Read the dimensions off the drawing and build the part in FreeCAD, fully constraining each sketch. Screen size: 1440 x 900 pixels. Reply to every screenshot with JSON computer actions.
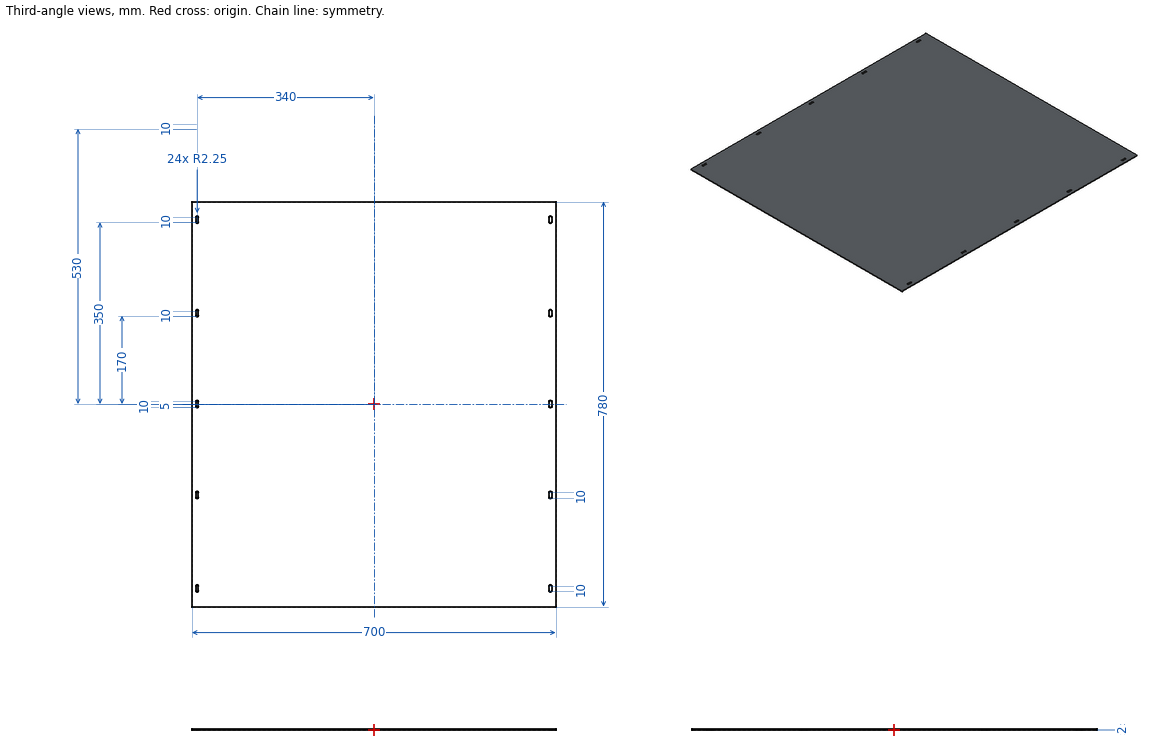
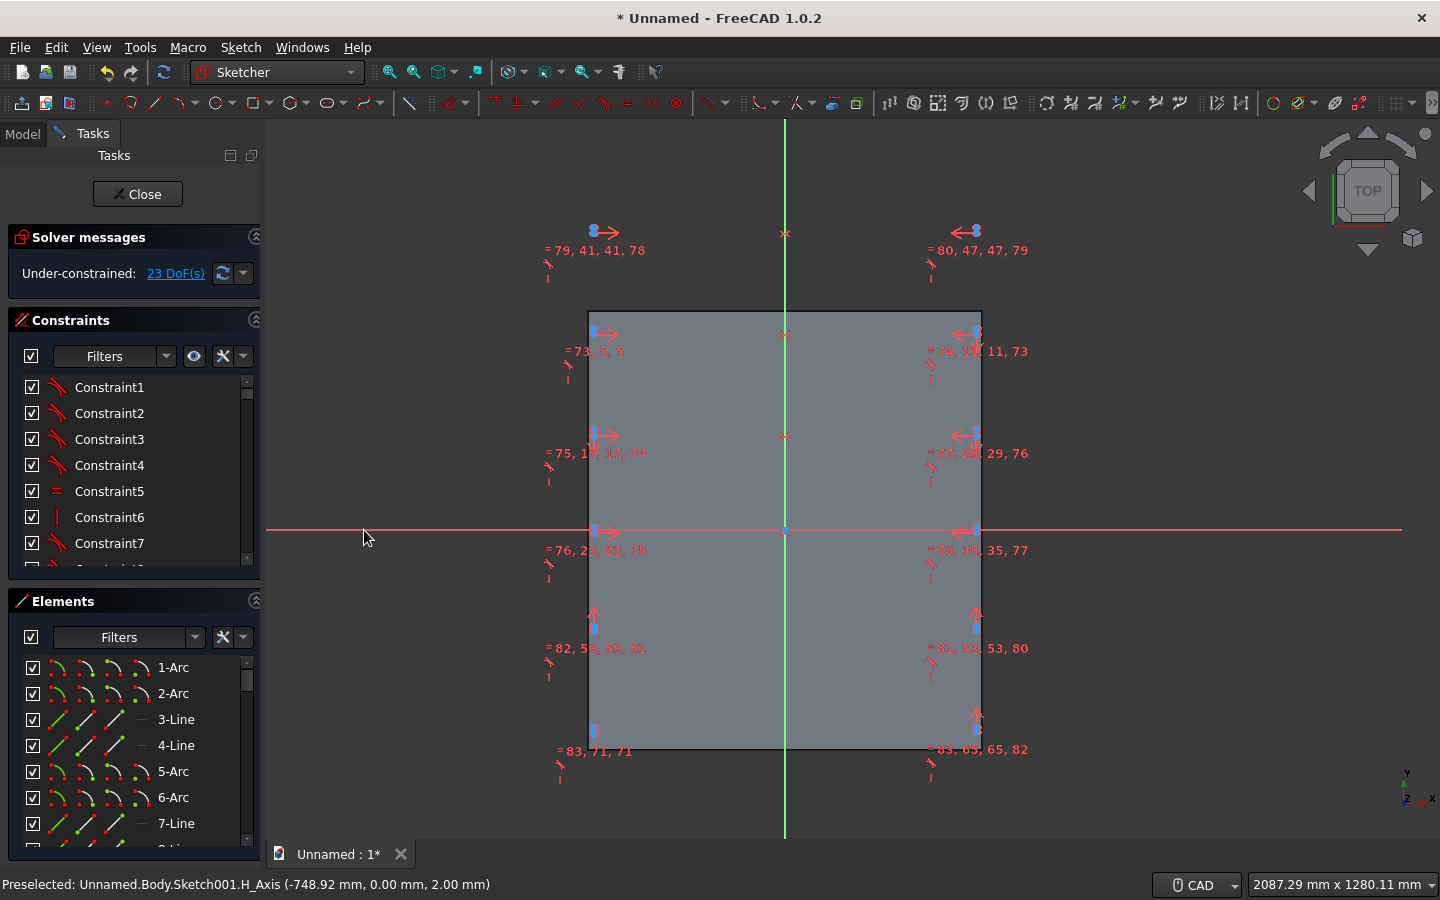
{"action": "scroll", "coordinate": [594, 328], "scroll_direction": "up", "scroll_amount": 12}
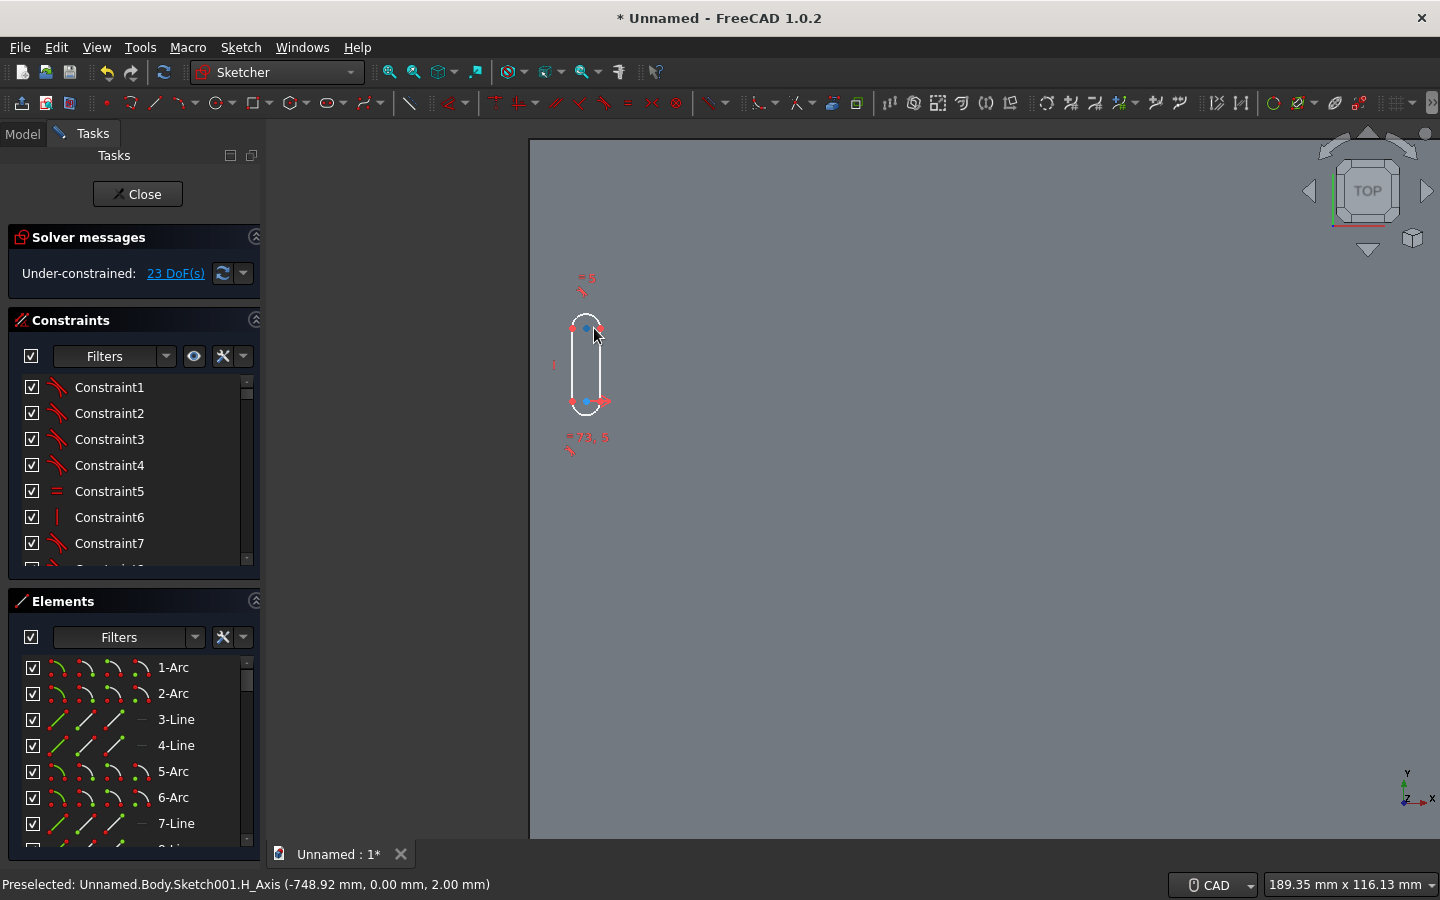
{"action": "left_click", "coordinate": [586, 328]}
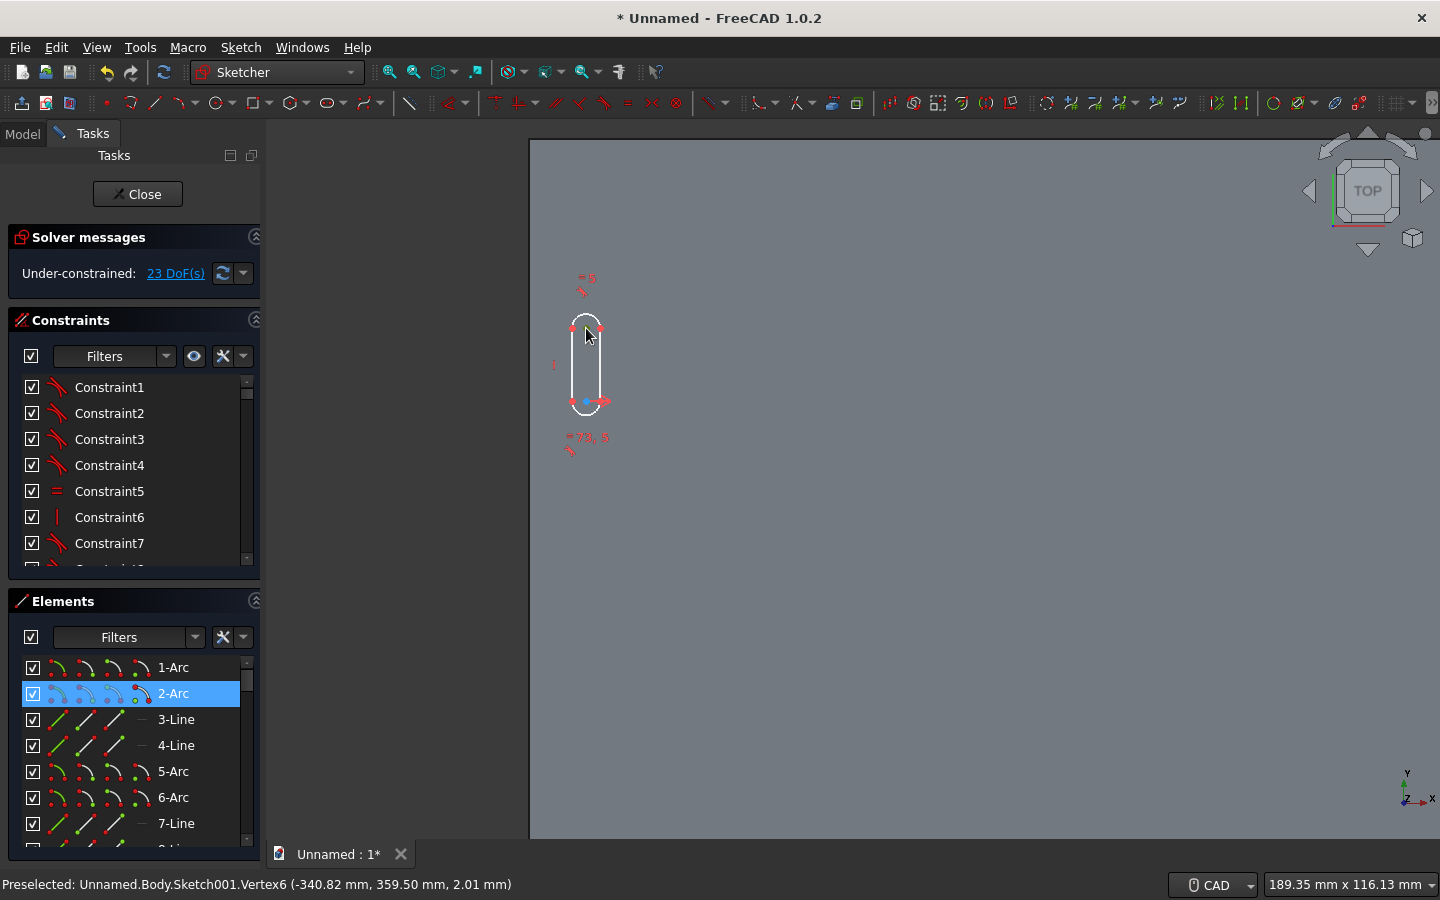
{"action": "scroll", "coordinate": [593, 327], "scroll_direction": "down", "scroll_amount": 12}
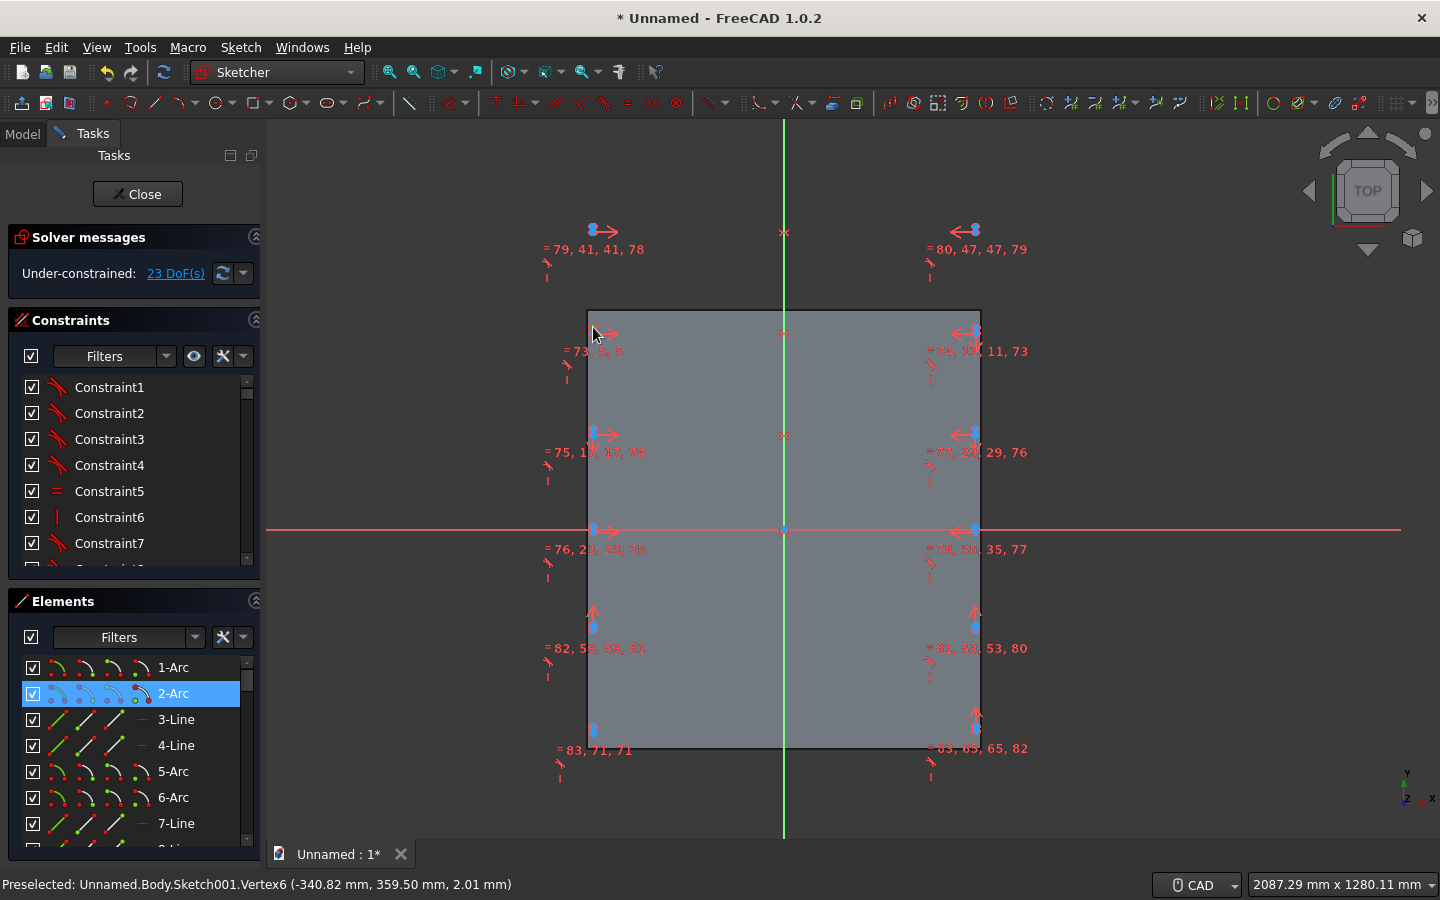
{"action": "scroll", "coordinate": [593, 733], "scroll_direction": "up", "scroll_amount": 12}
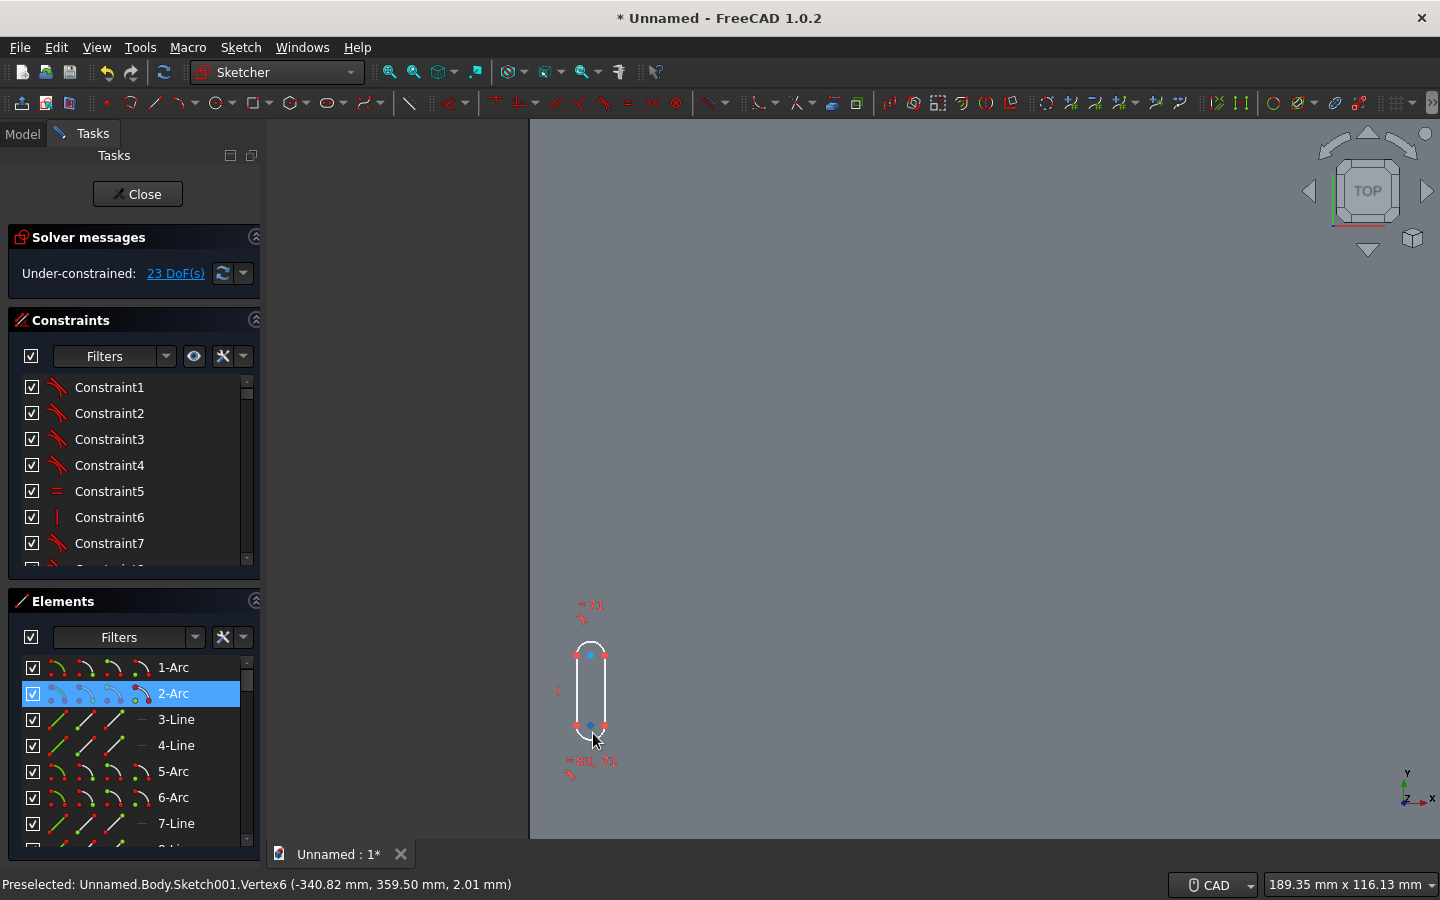
{"action": "left_click", "coordinate": [591, 726]}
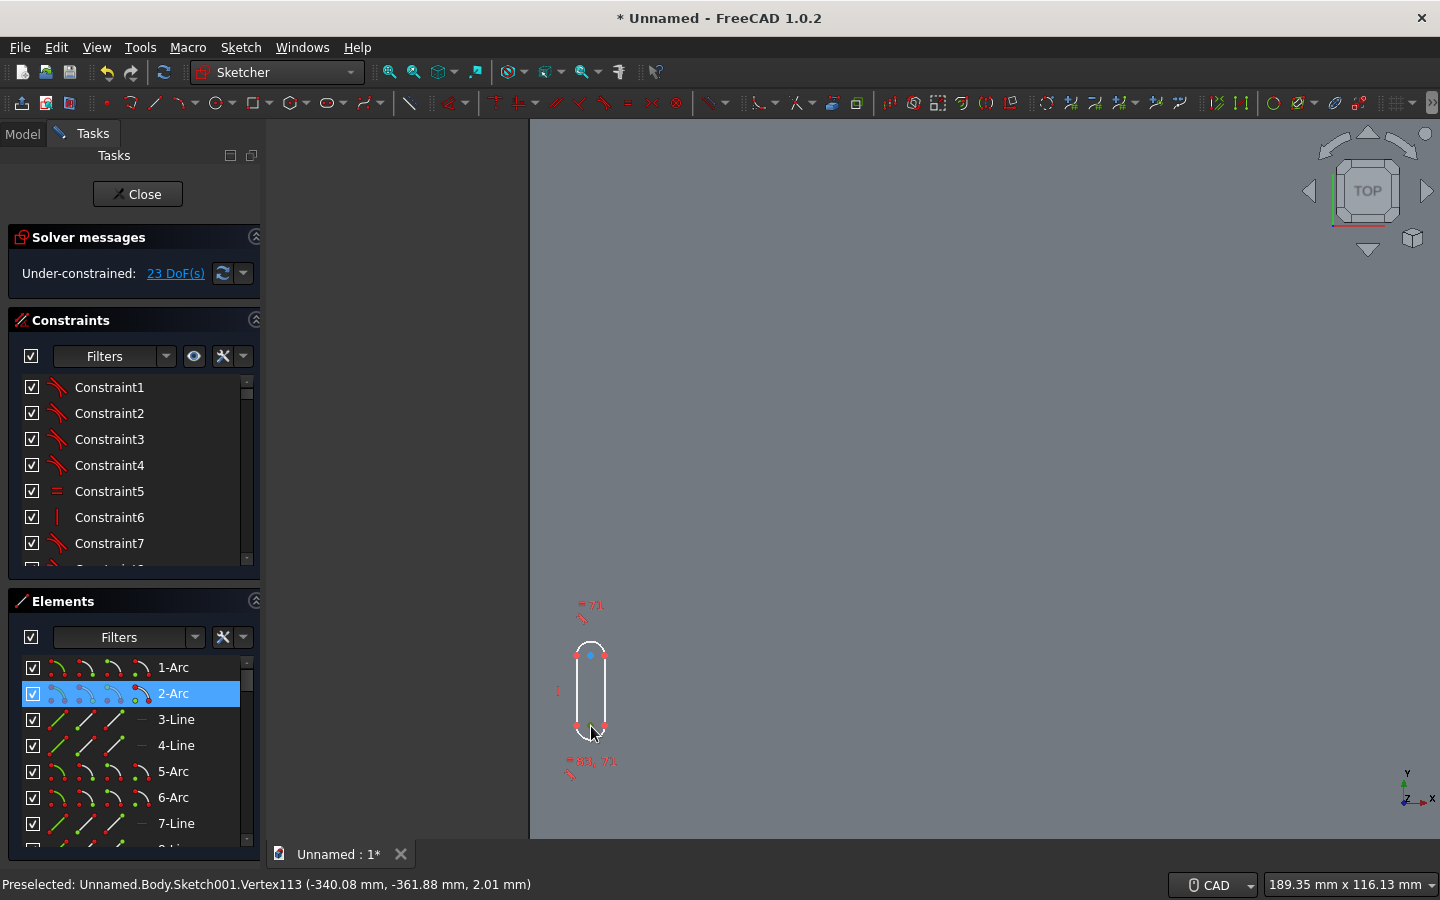
{"action": "scroll", "coordinate": [593, 734], "scroll_direction": "down", "scroll_amount": 12}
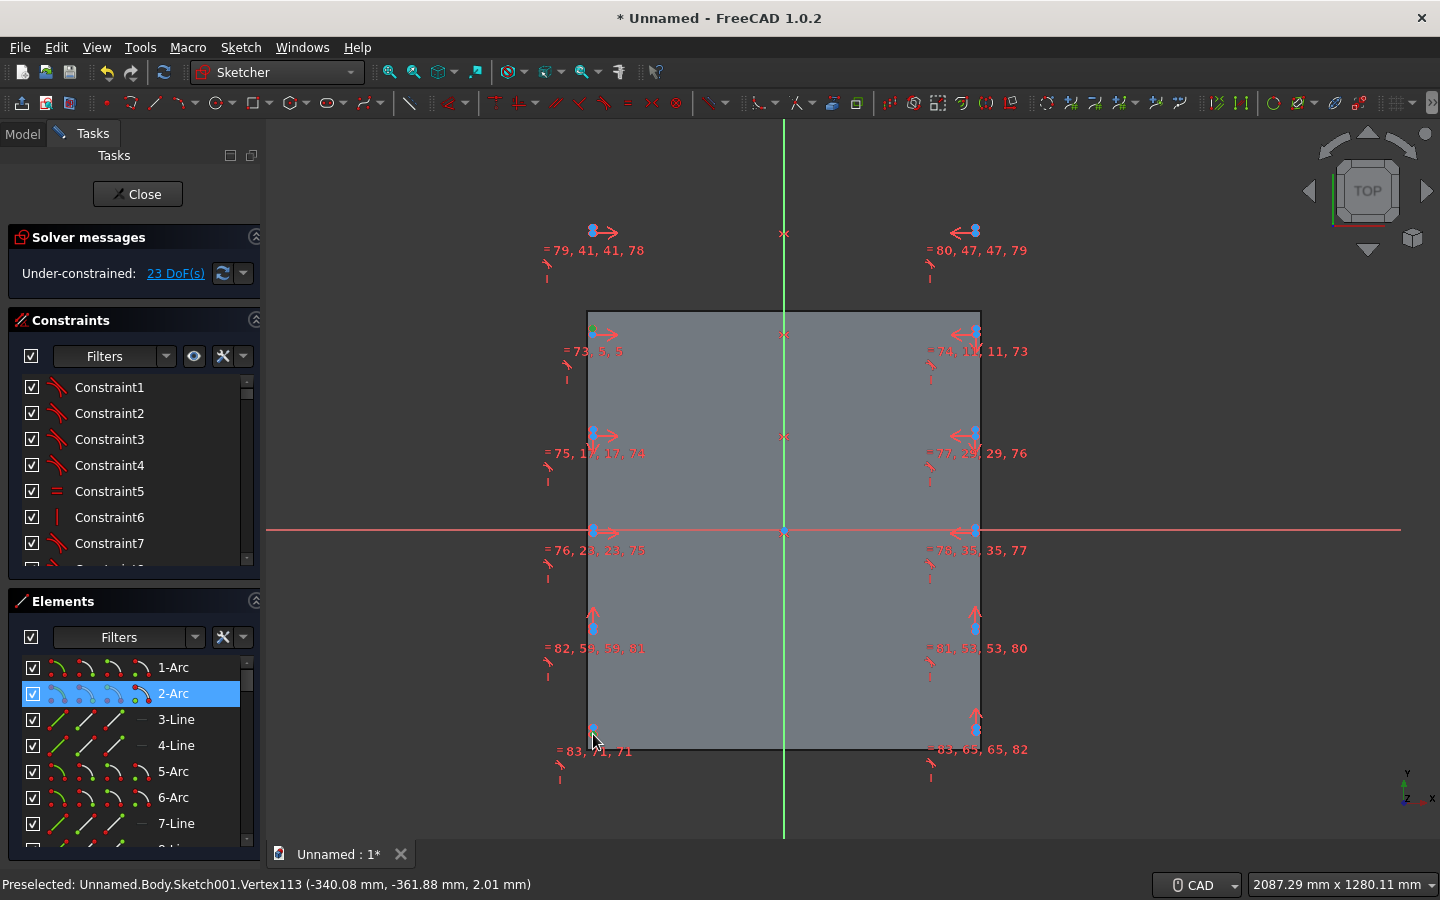
{"action": "left_click", "coordinate": [364, 530]}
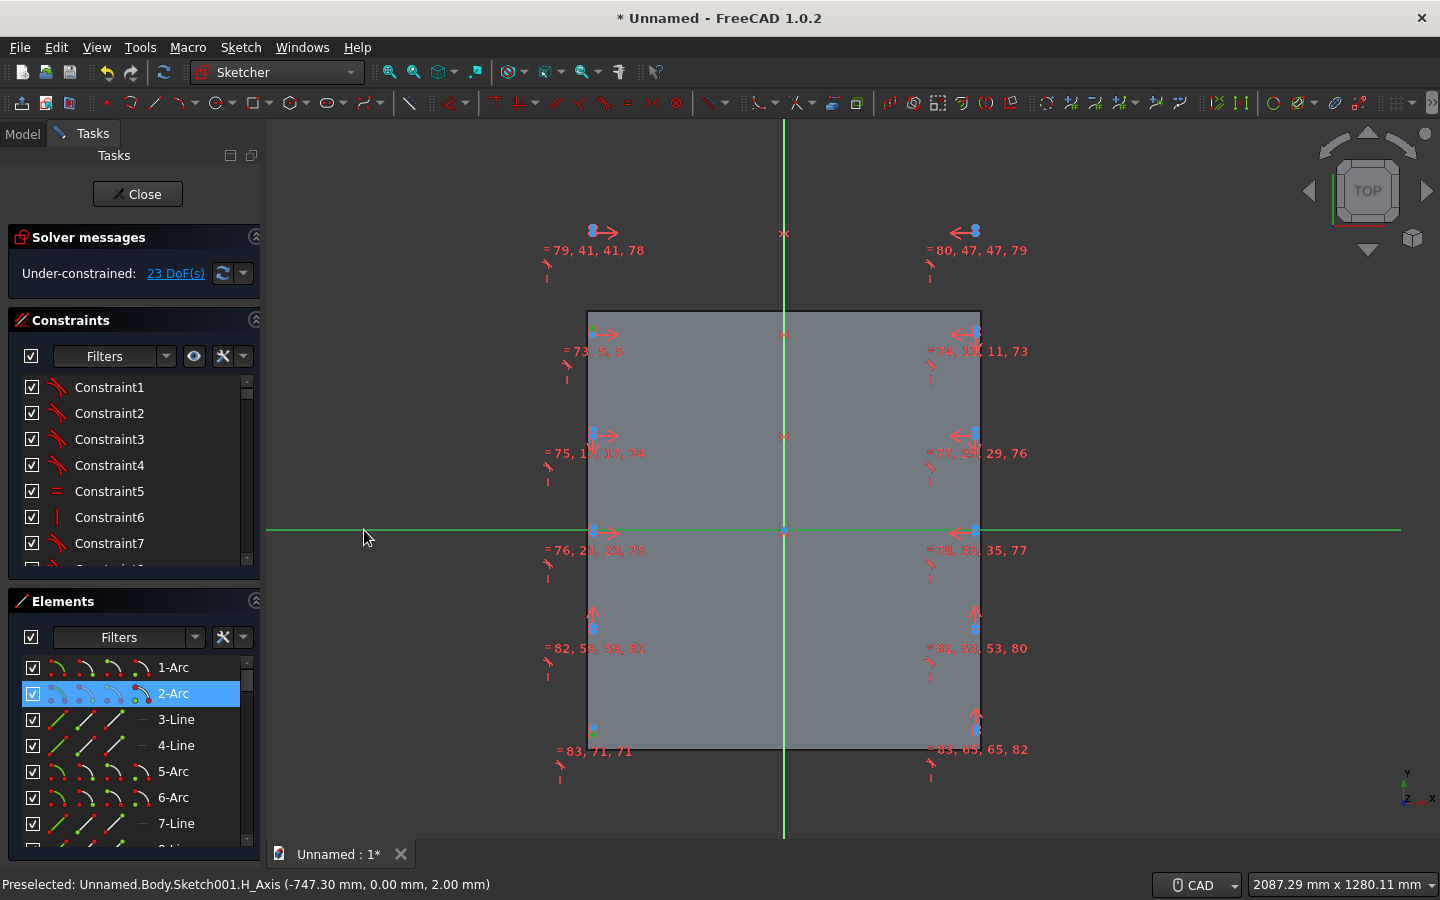
{"action": "key", "text": "s"}